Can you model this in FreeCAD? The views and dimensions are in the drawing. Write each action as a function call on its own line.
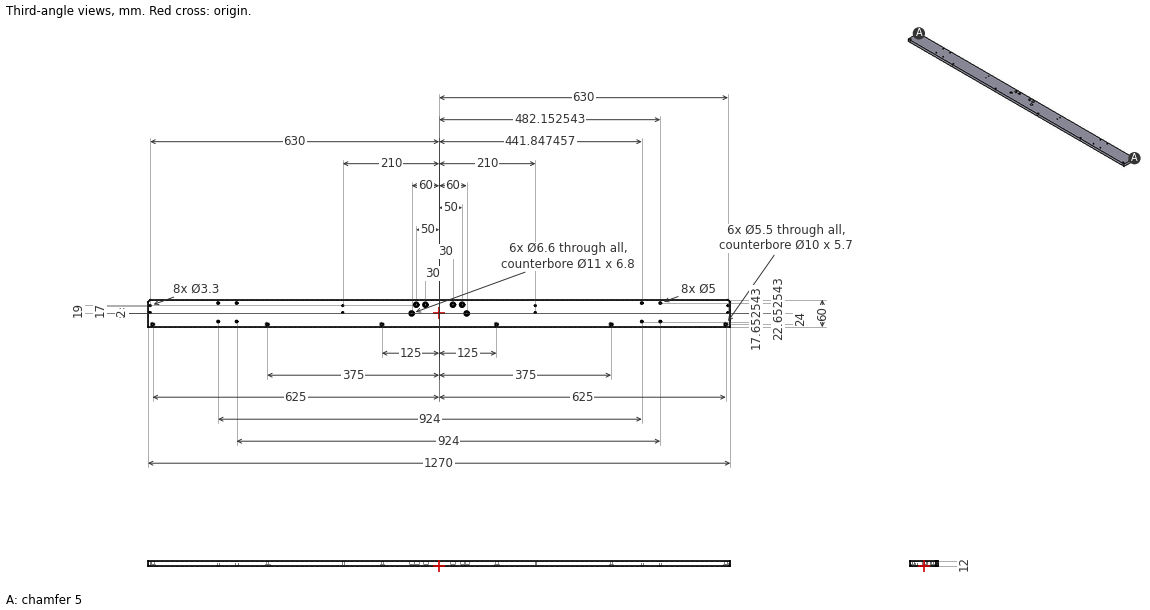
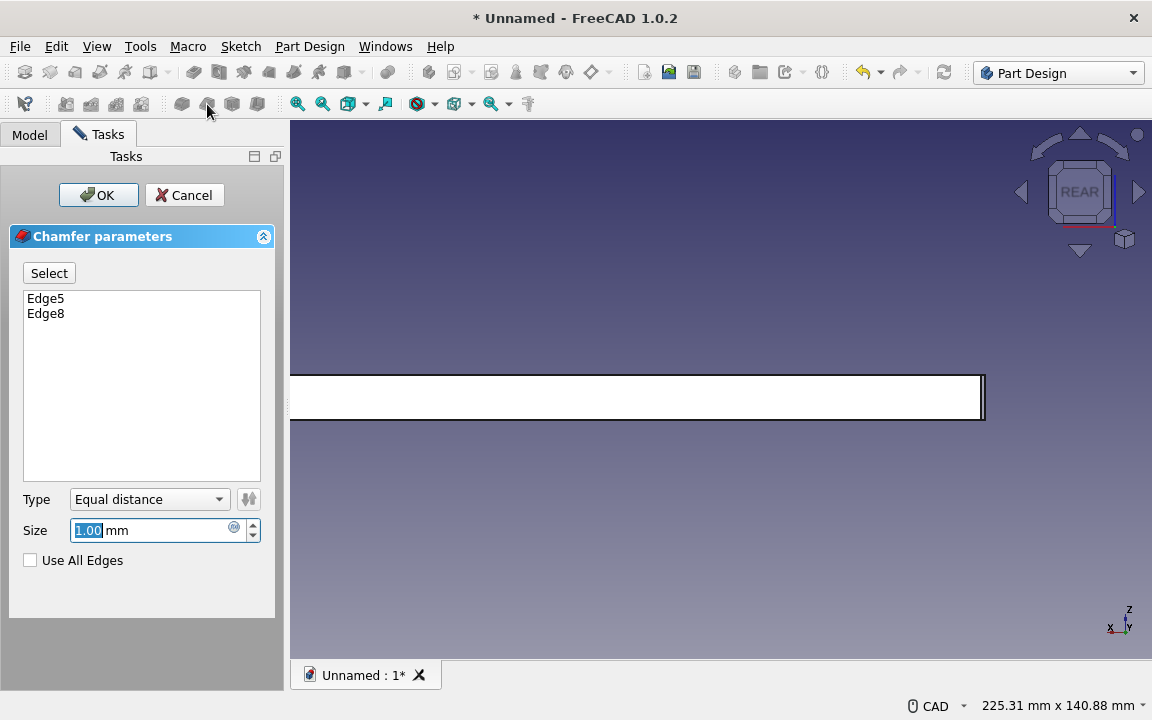
text(5)
key(Tab)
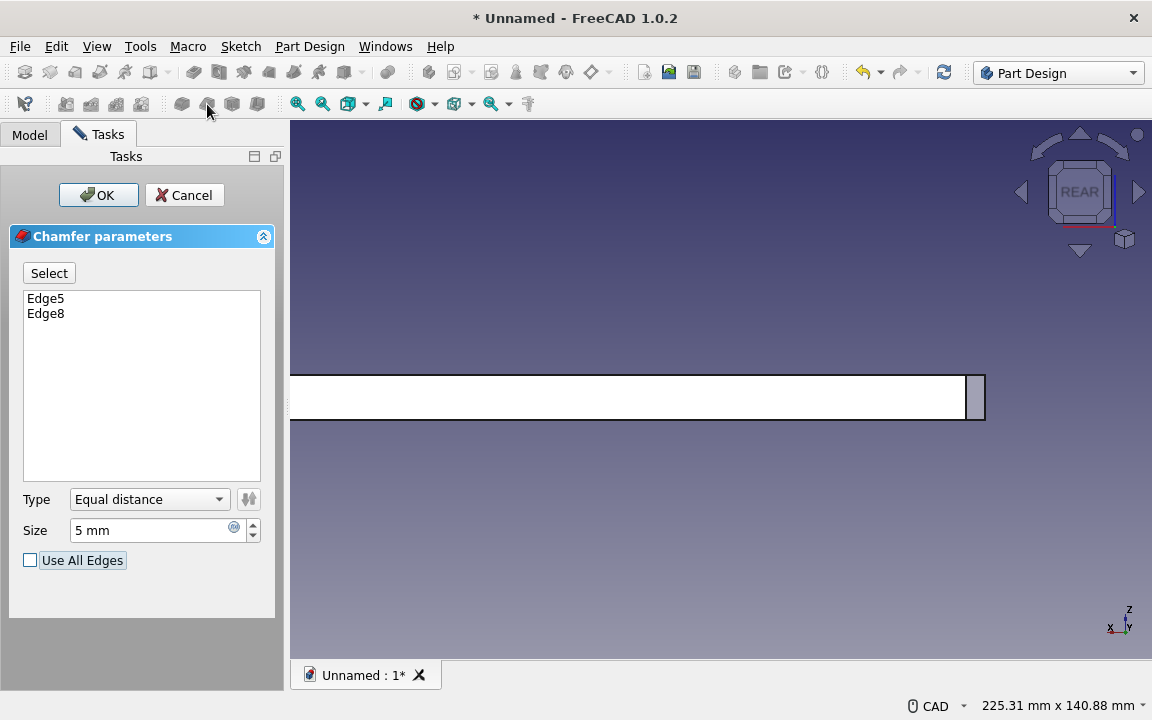
click(99, 195)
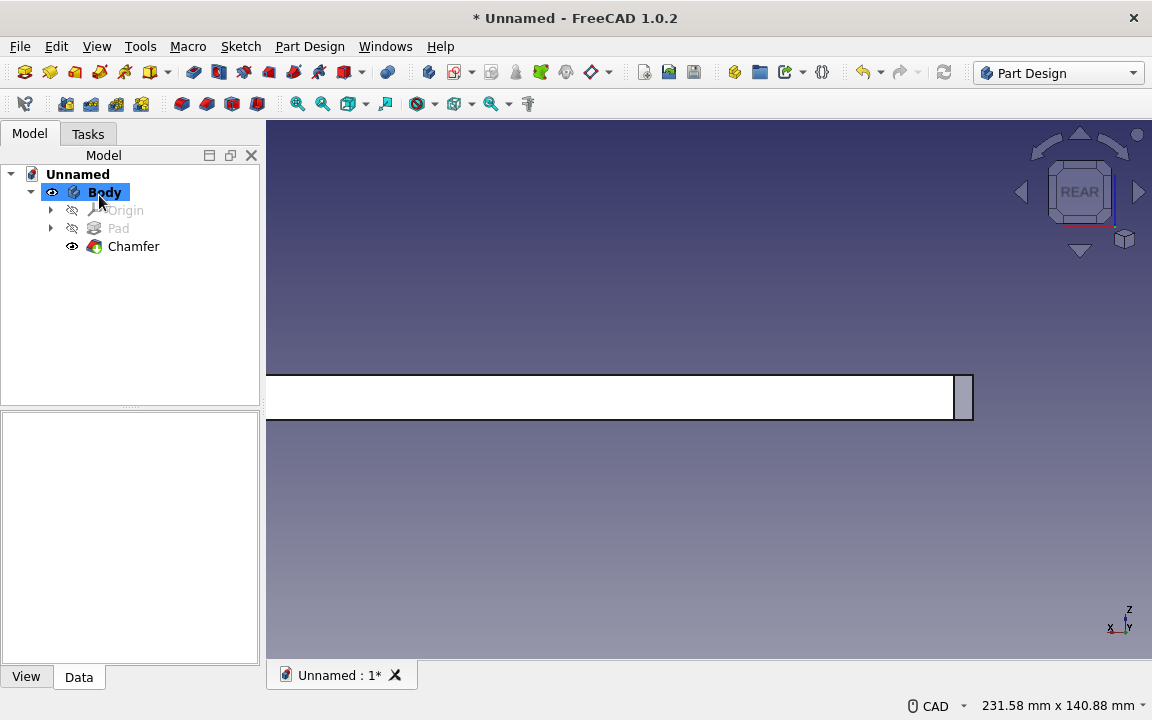
click(298, 104)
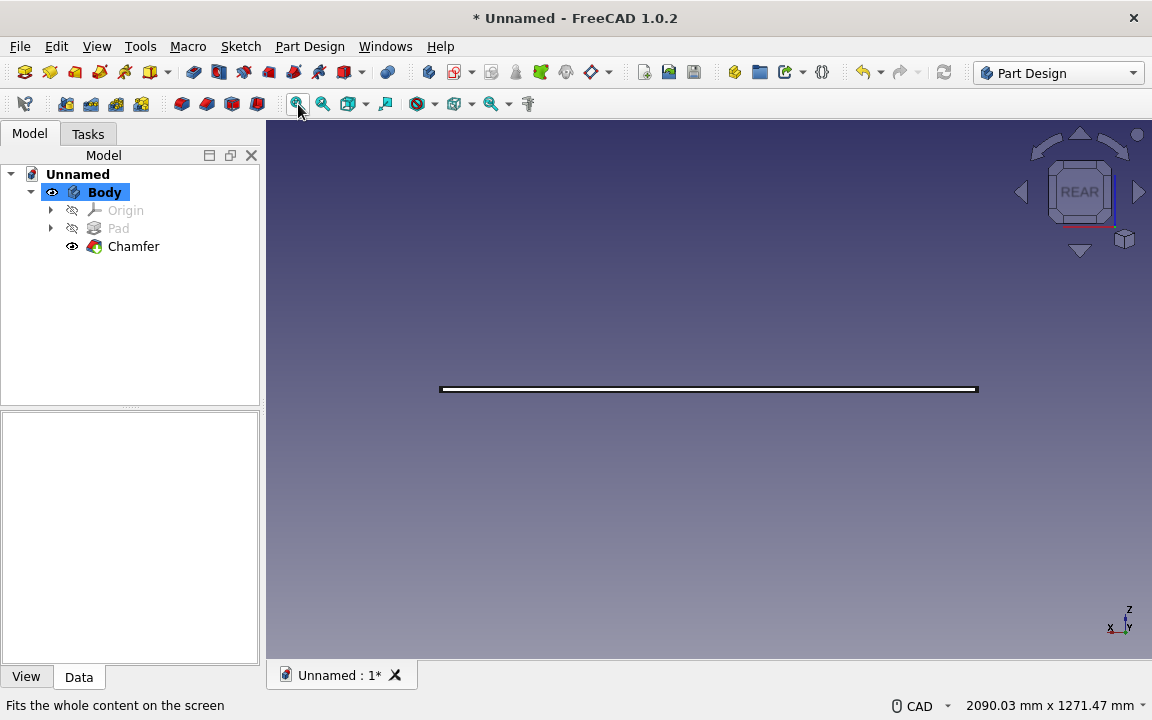
key(5)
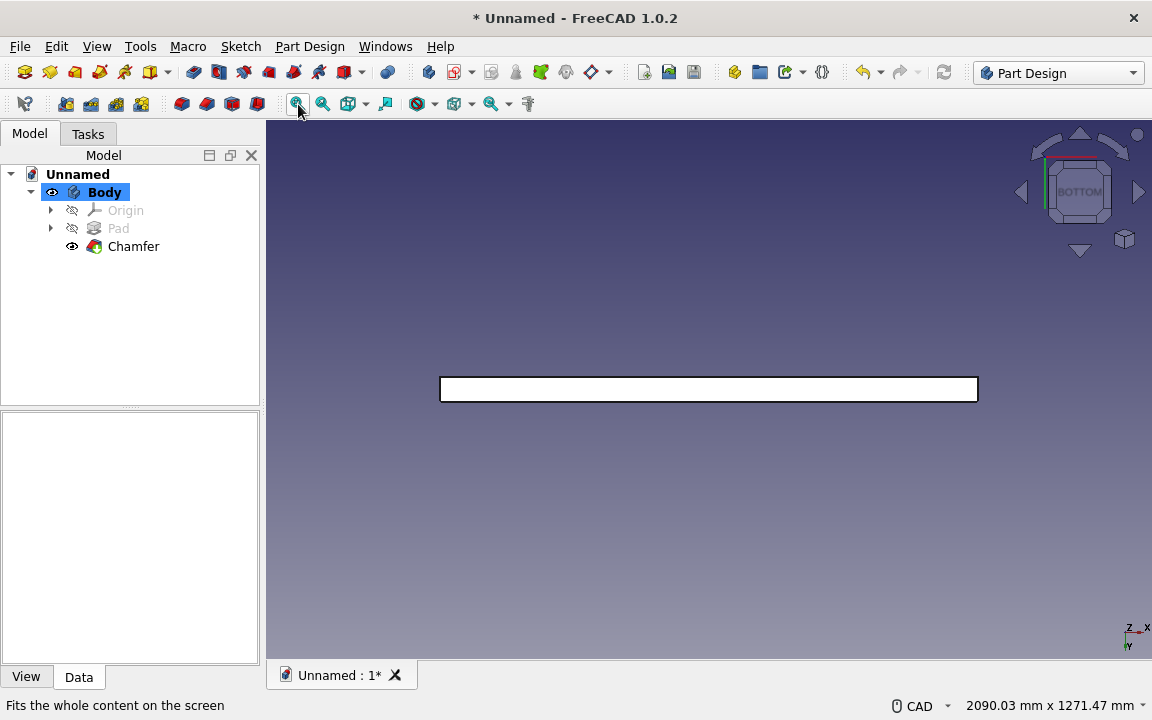
click(940, 388)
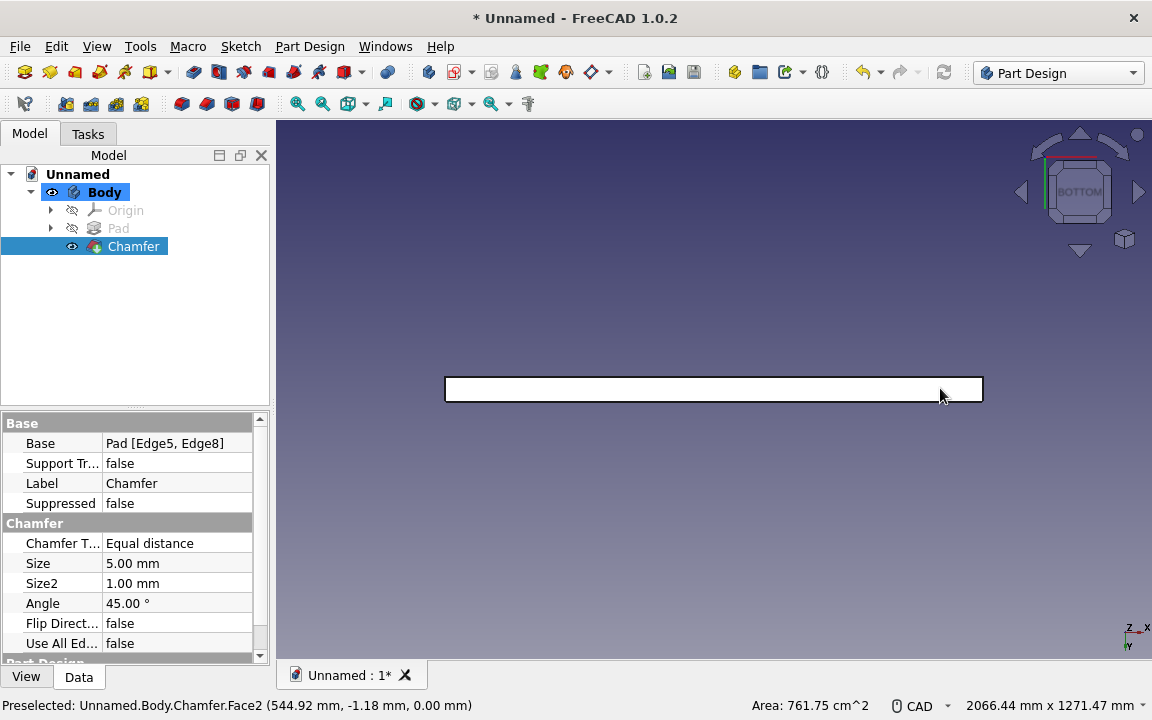
click(454, 72)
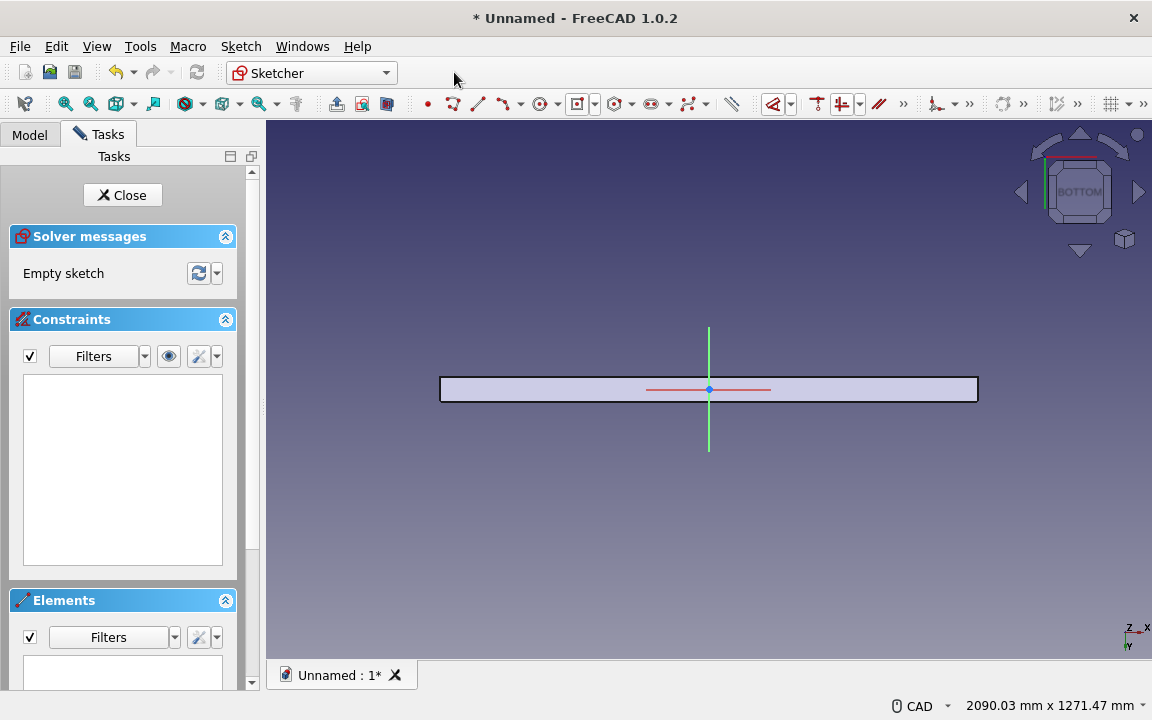
scroll(331, 415, down, 1)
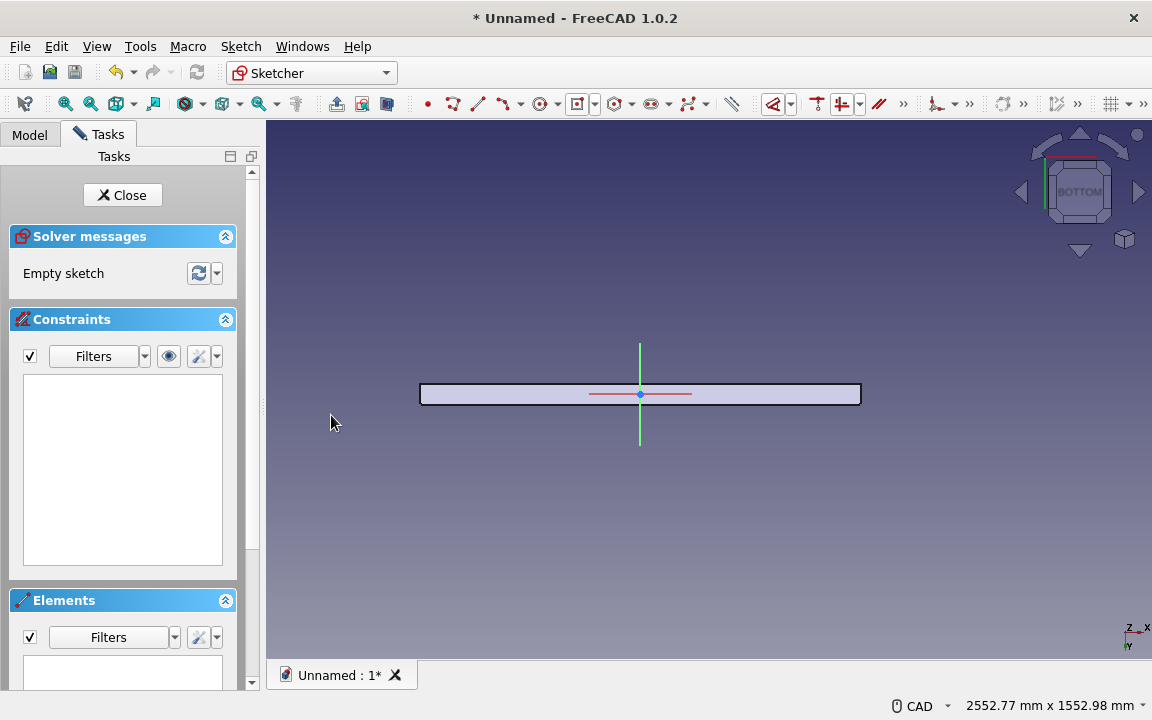
key(g)
key(c)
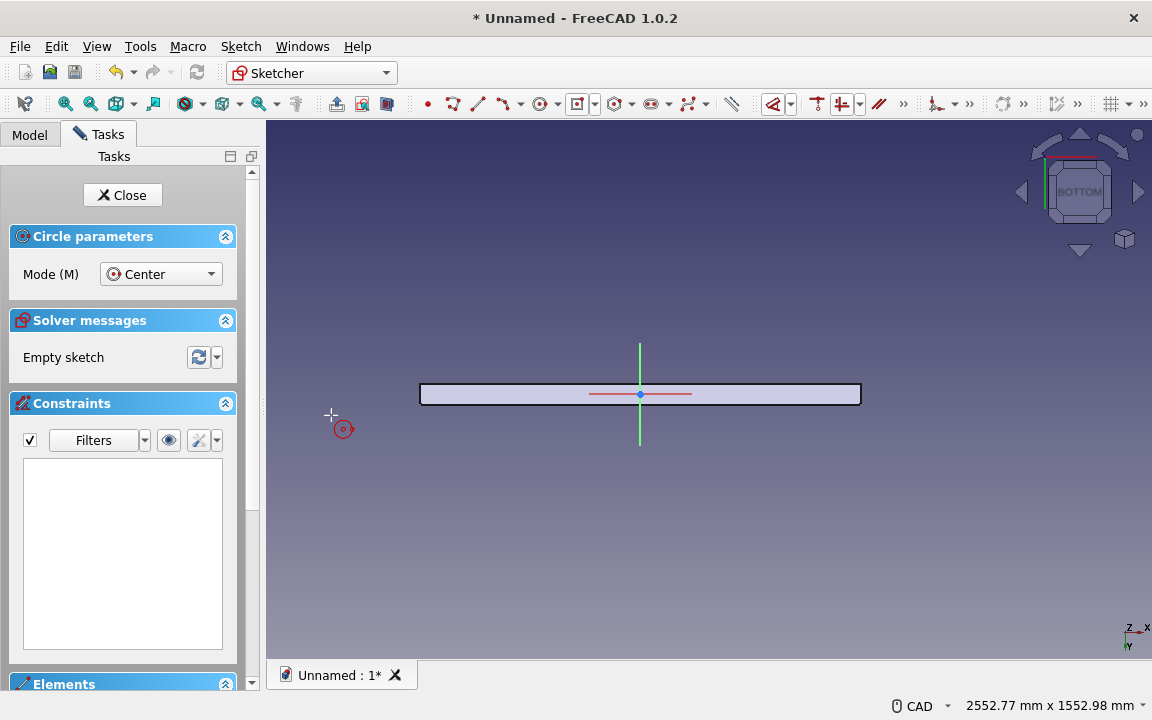
scroll(857, 386, up, 16)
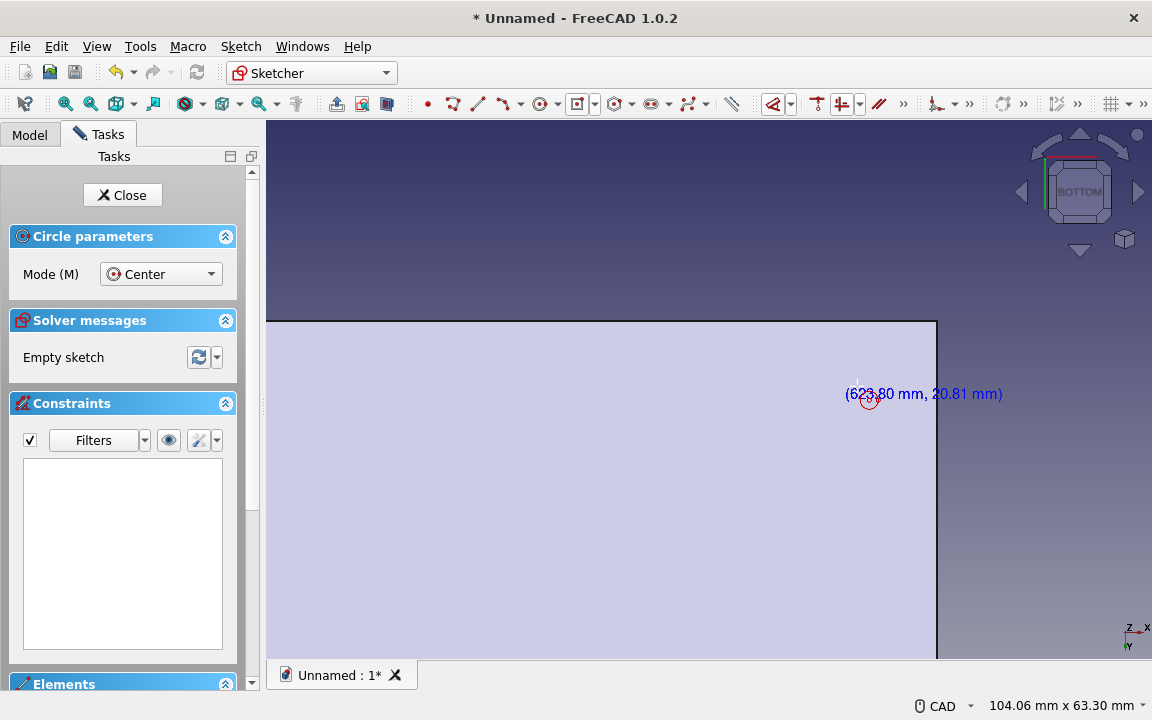
scroll(908, 386, down, 15)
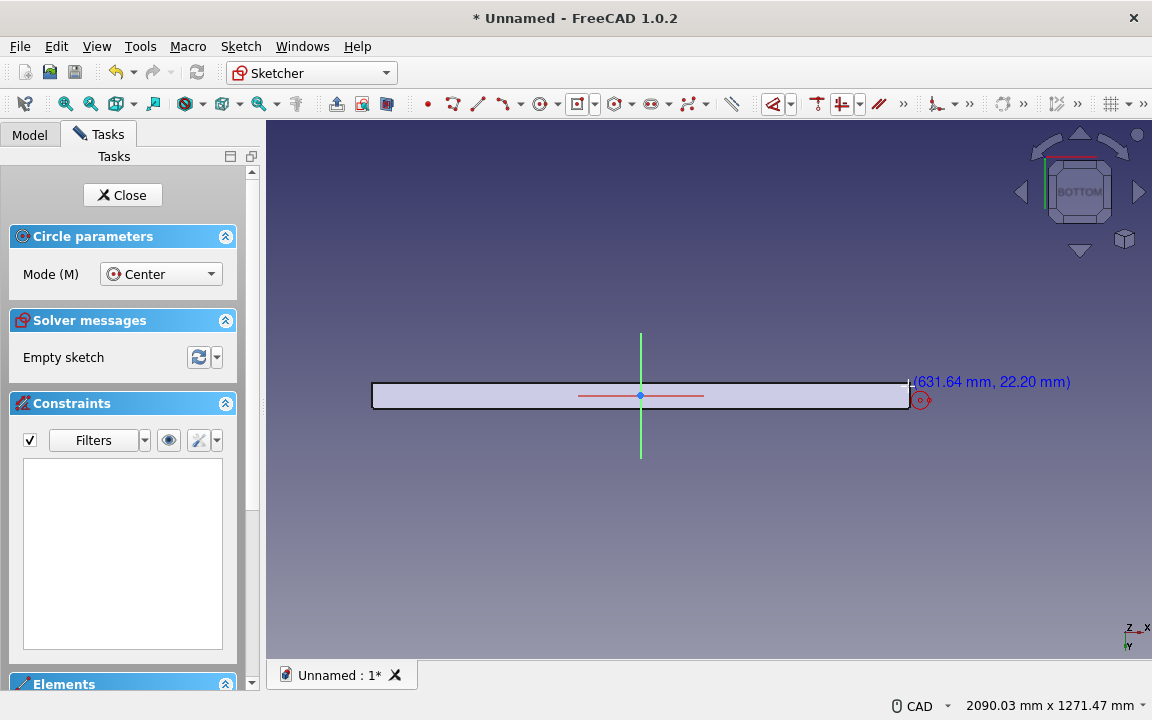
scroll(906, 386, up, 3)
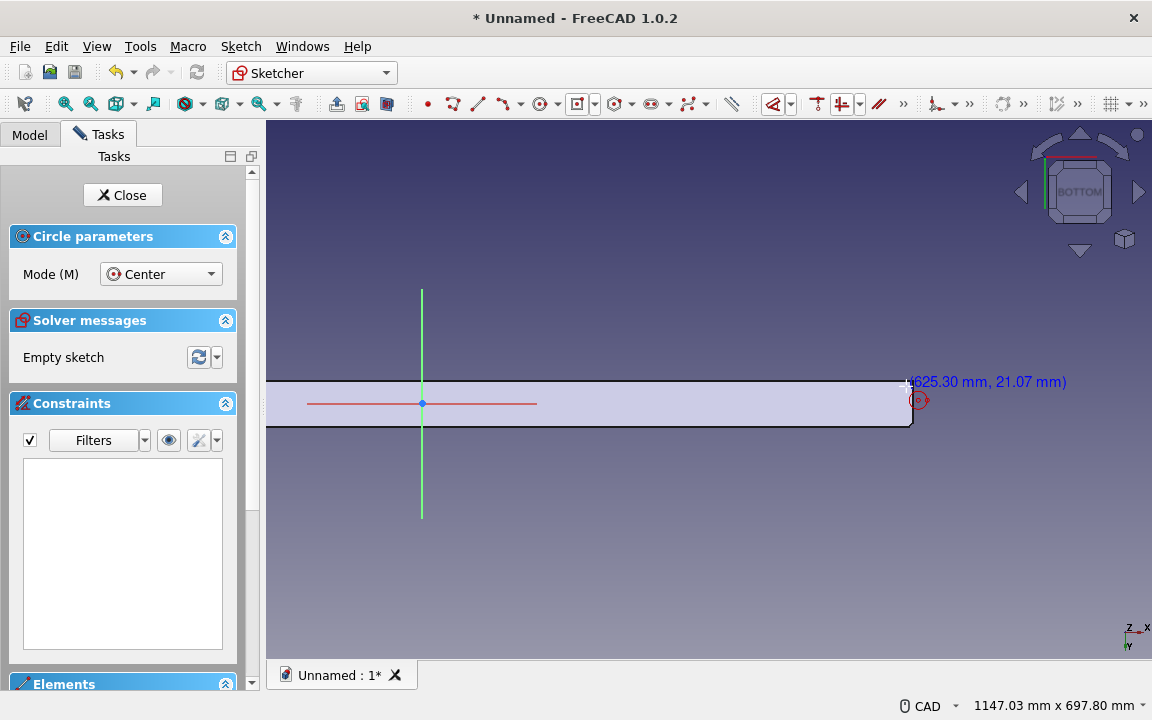
click(905, 385)